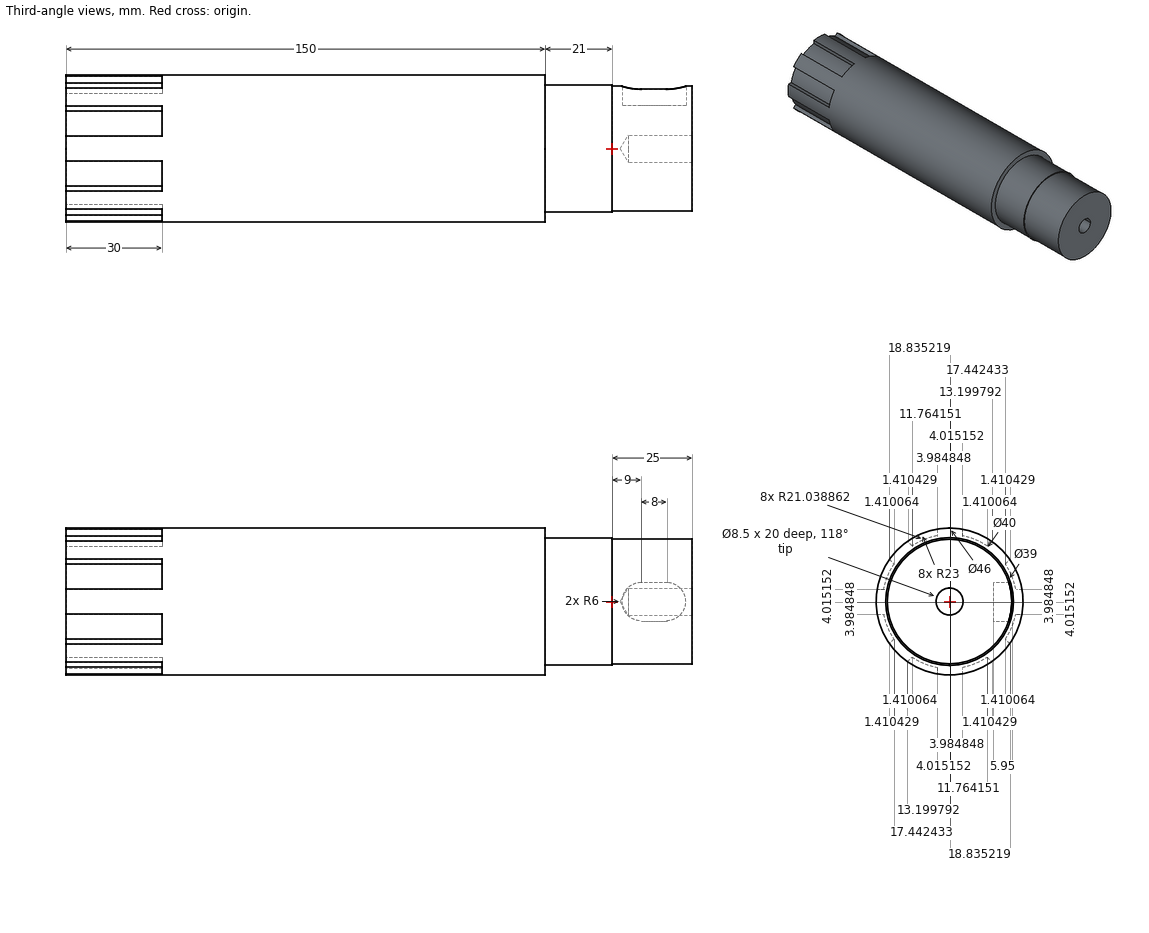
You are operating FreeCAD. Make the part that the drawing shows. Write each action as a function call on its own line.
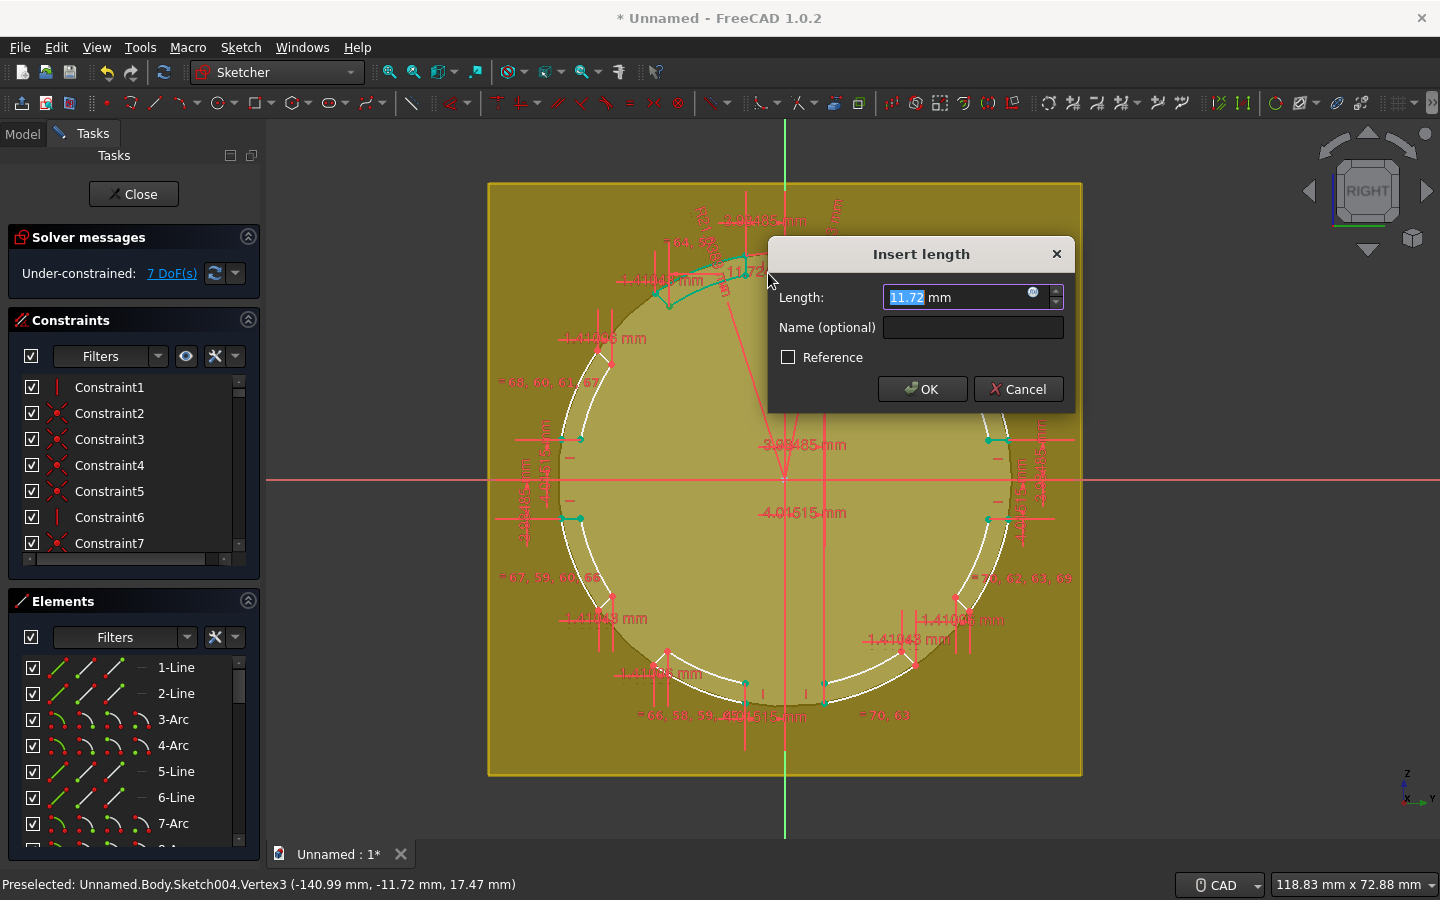
text(11.764151)
key(Return)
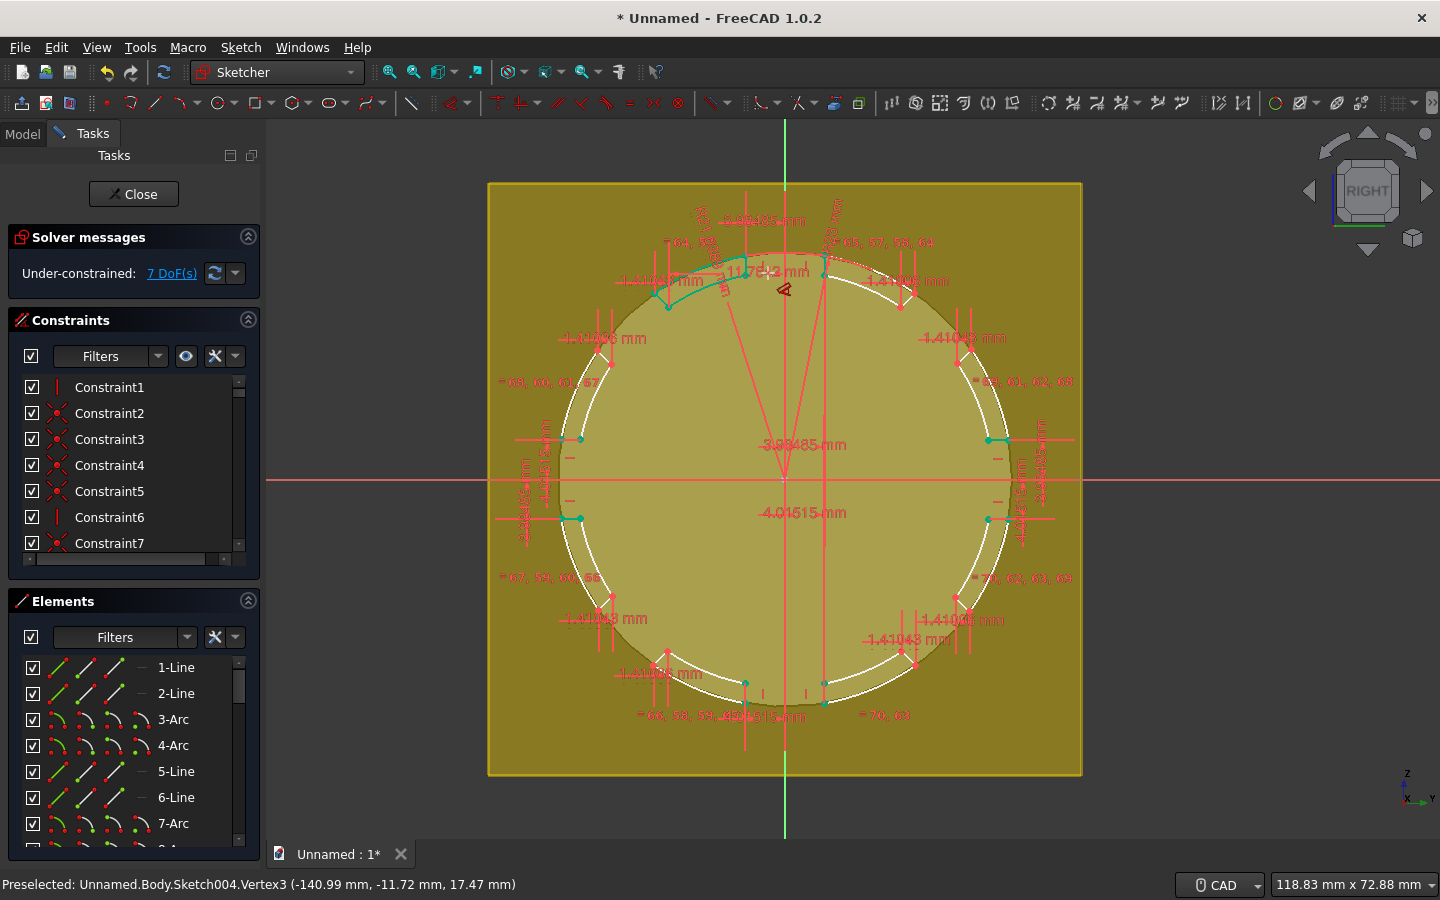
click(915, 293)
click(895, 259)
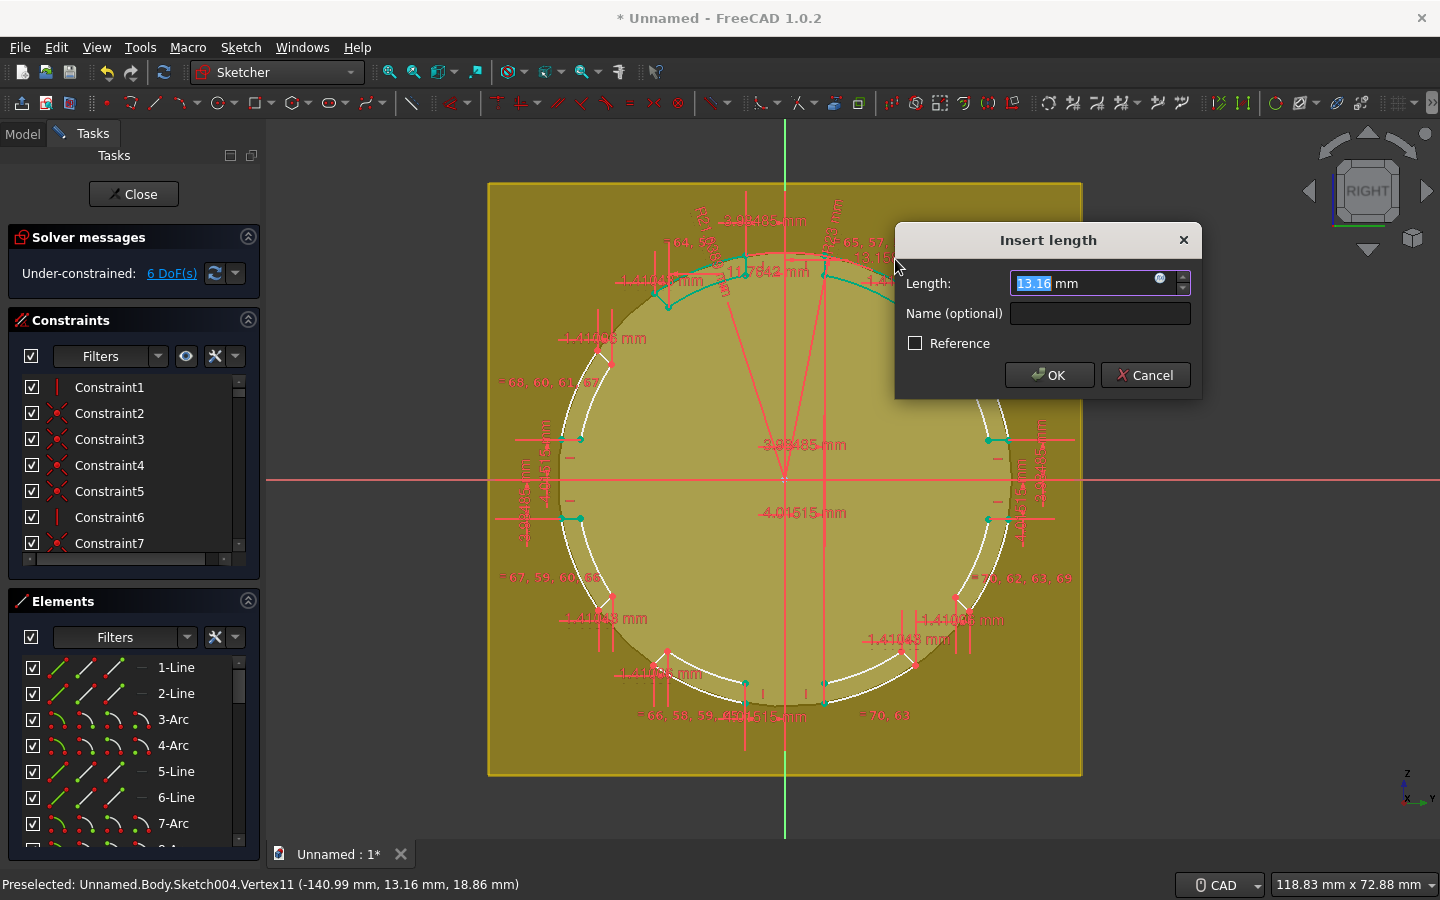
text(13.199792)
key(Return)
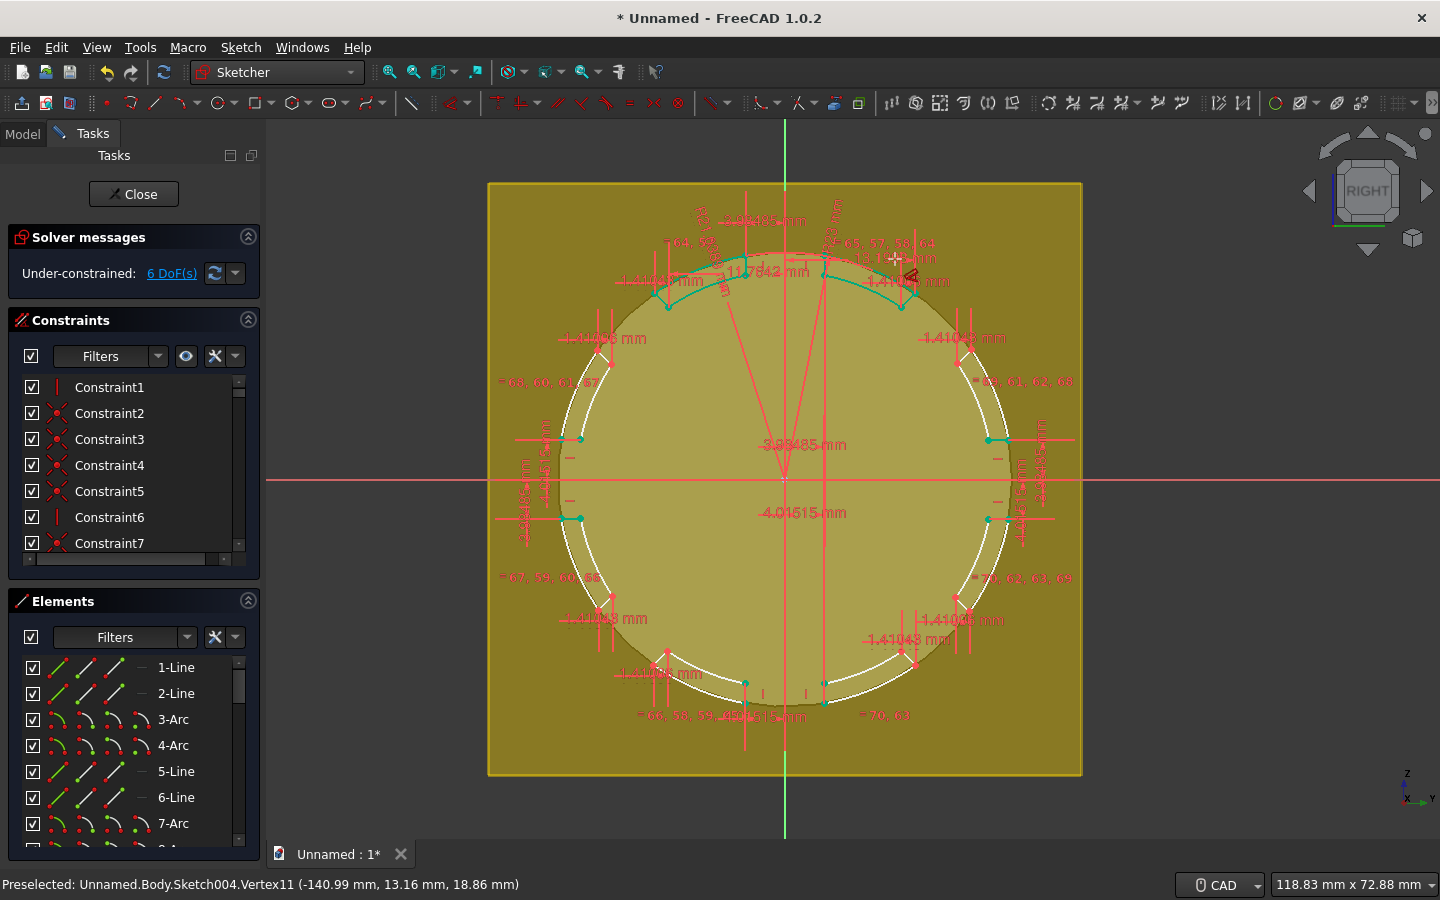
click(654, 665)
click(673, 699)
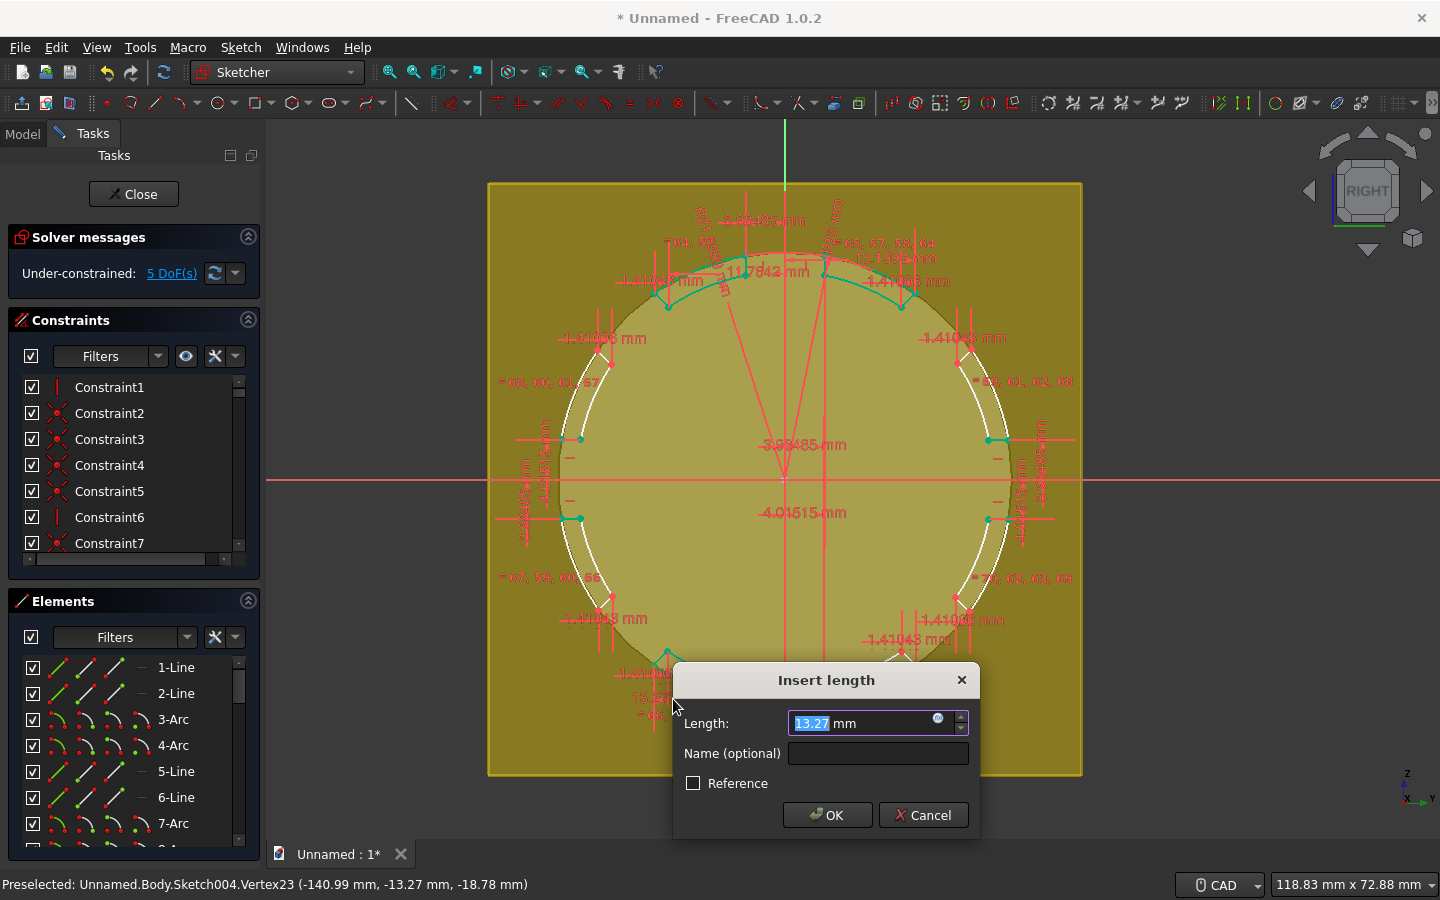
text(13.199792)
key(Return)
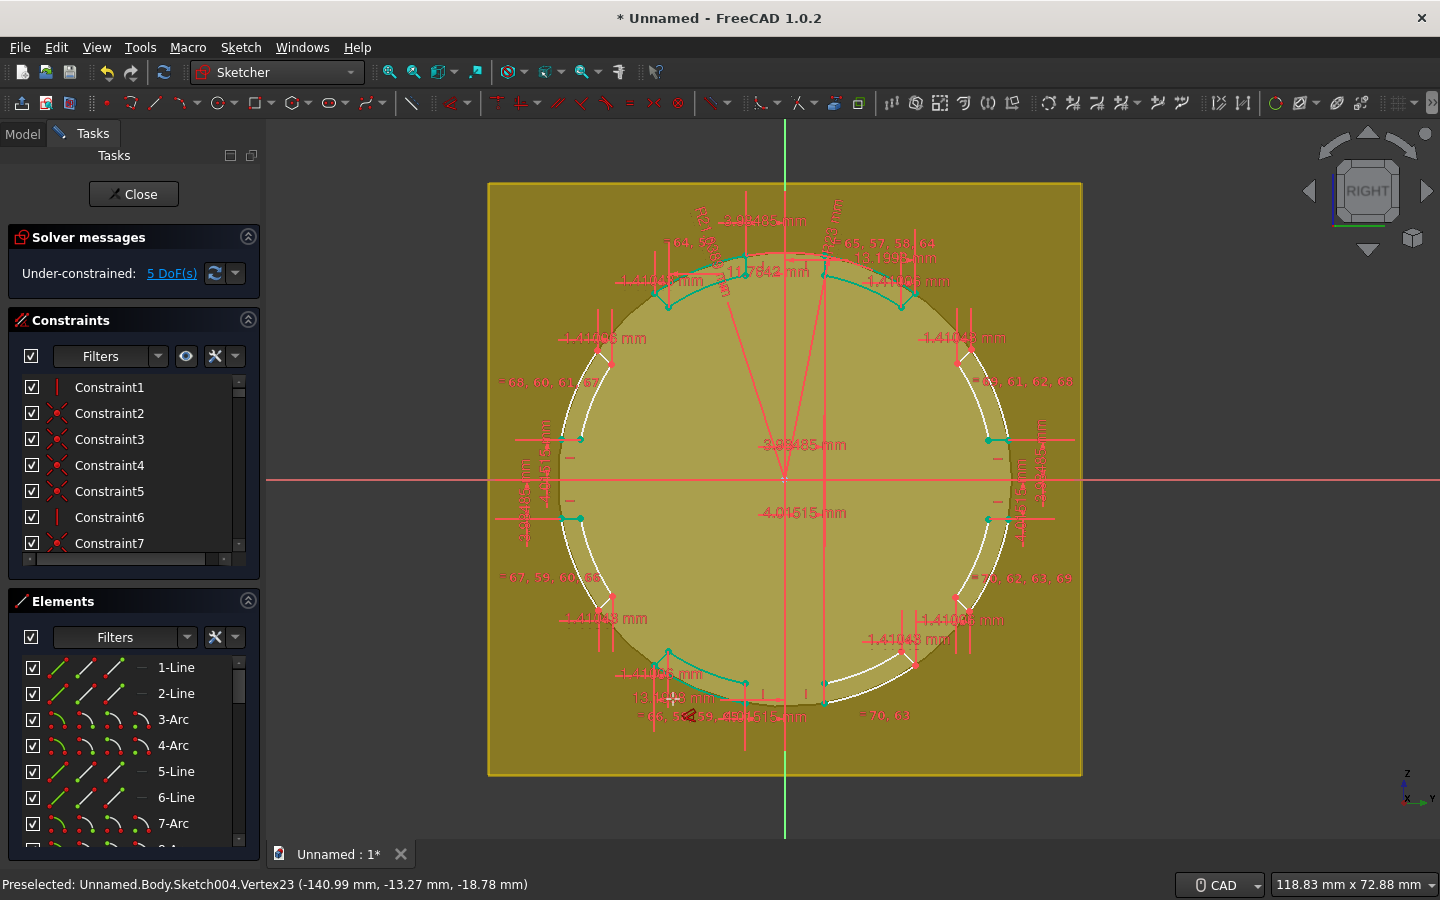
click(613, 596)
click(699, 630)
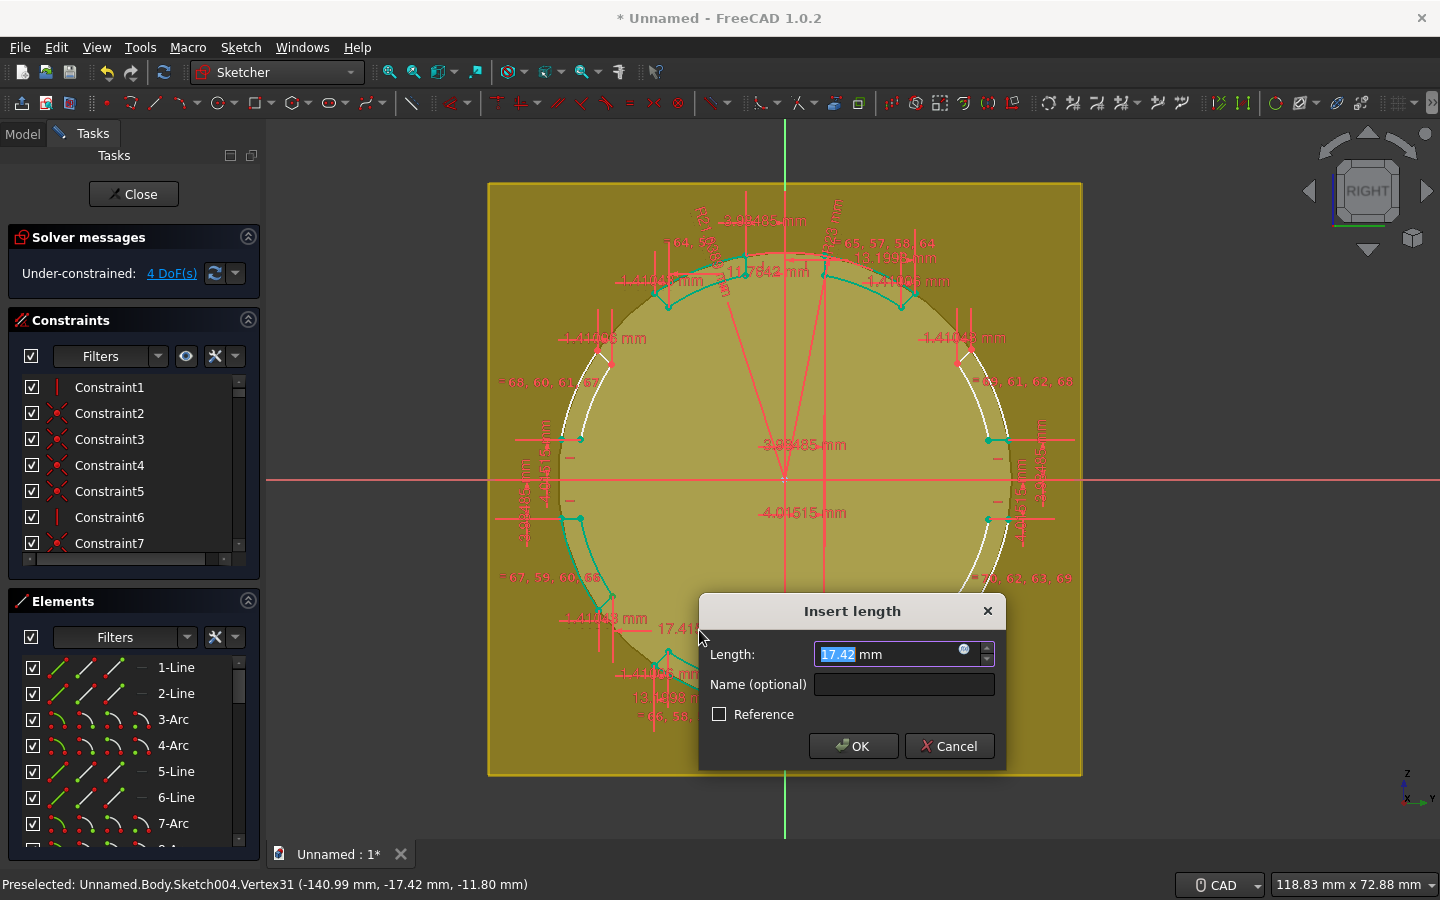
text(17.442433)
key(Return)